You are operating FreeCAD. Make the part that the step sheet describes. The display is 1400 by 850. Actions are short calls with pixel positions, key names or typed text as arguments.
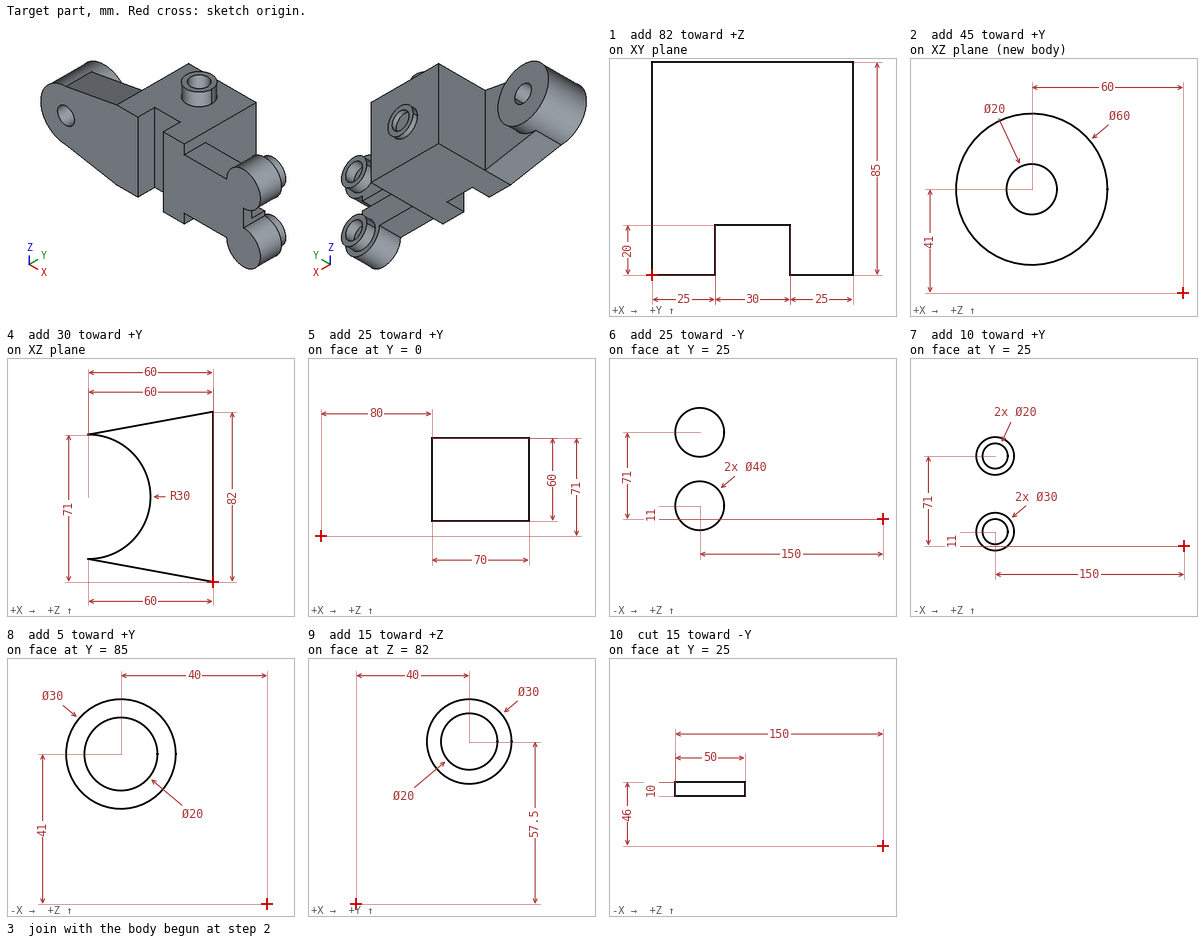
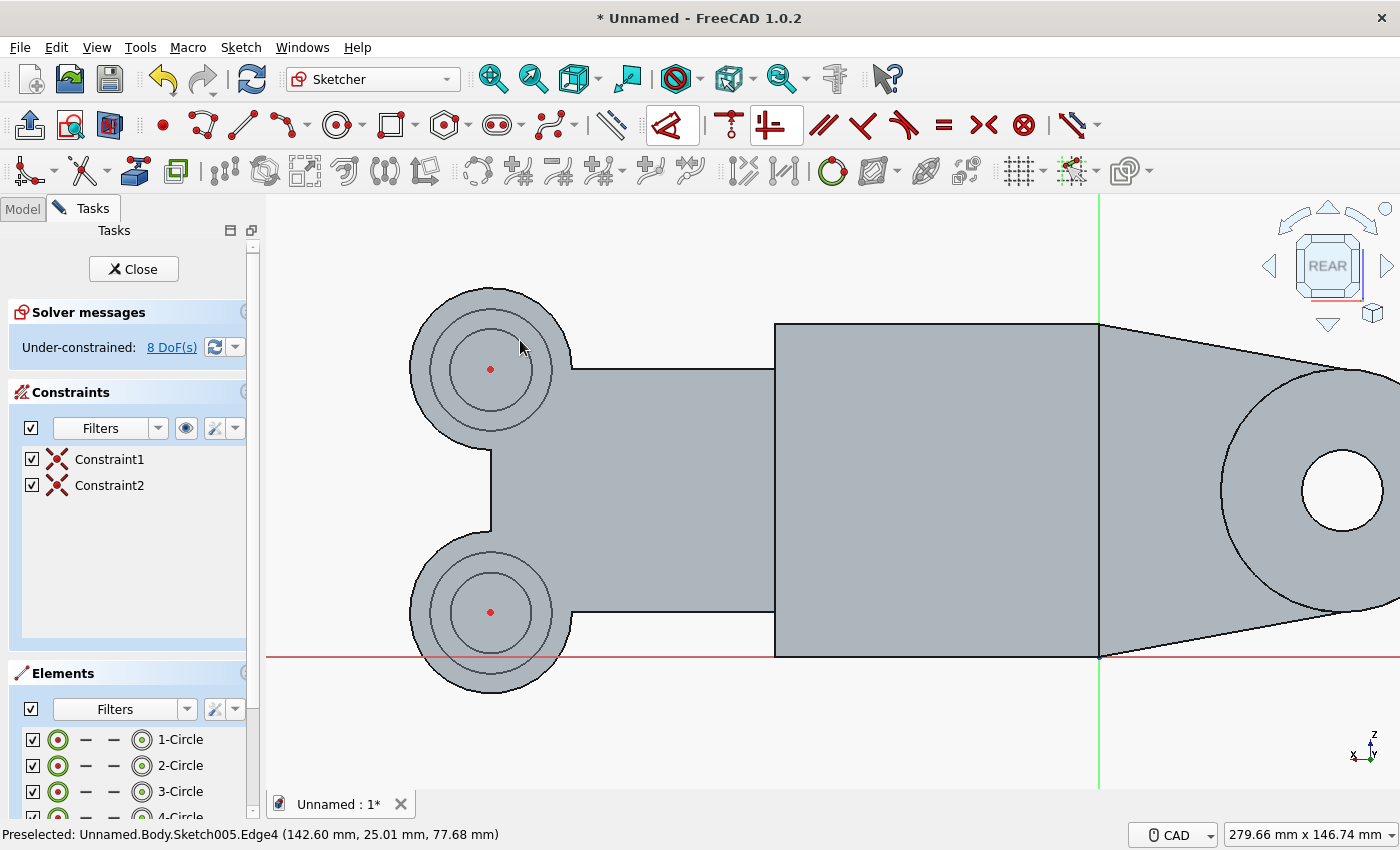
click(534, 570)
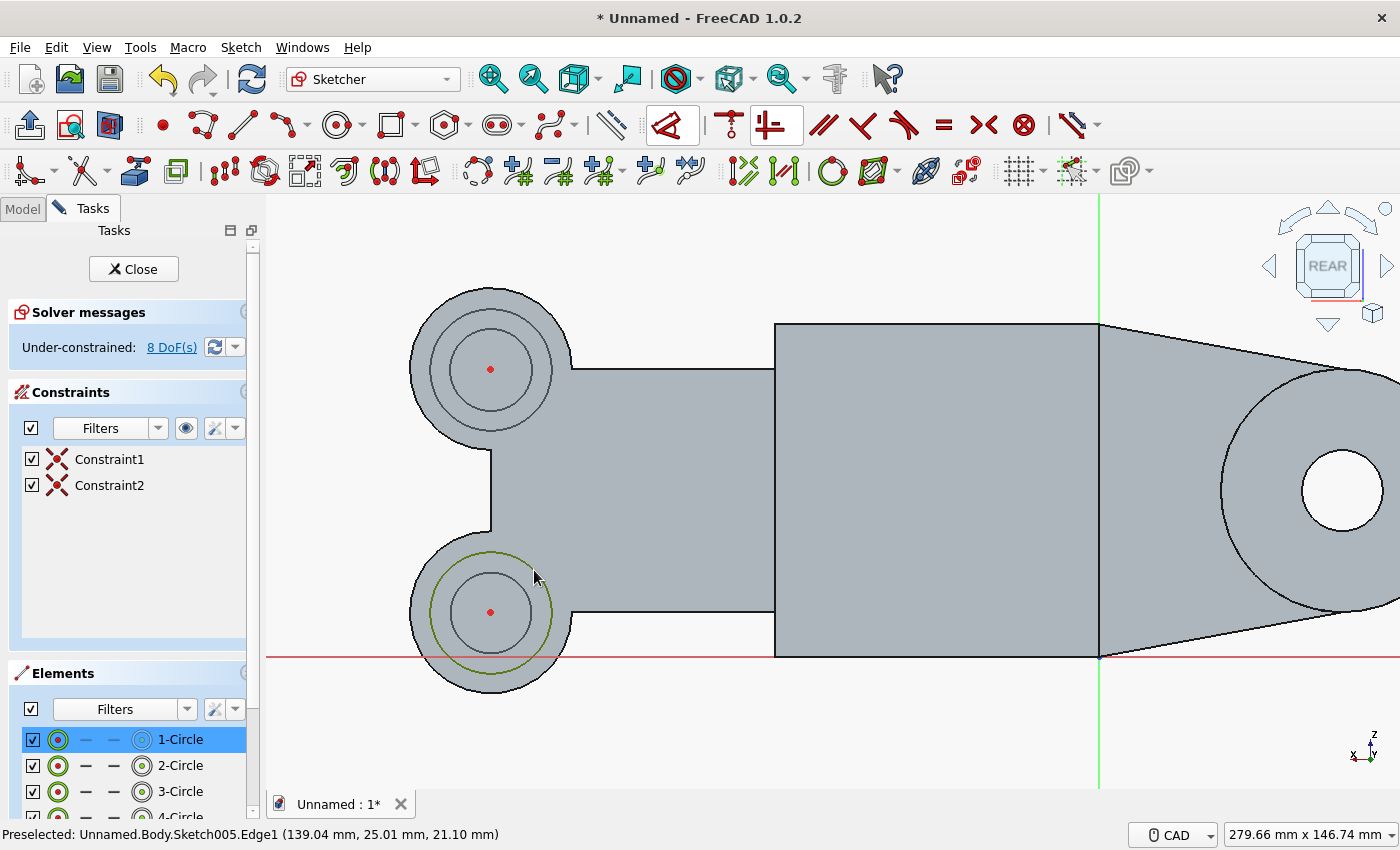
click(534, 327)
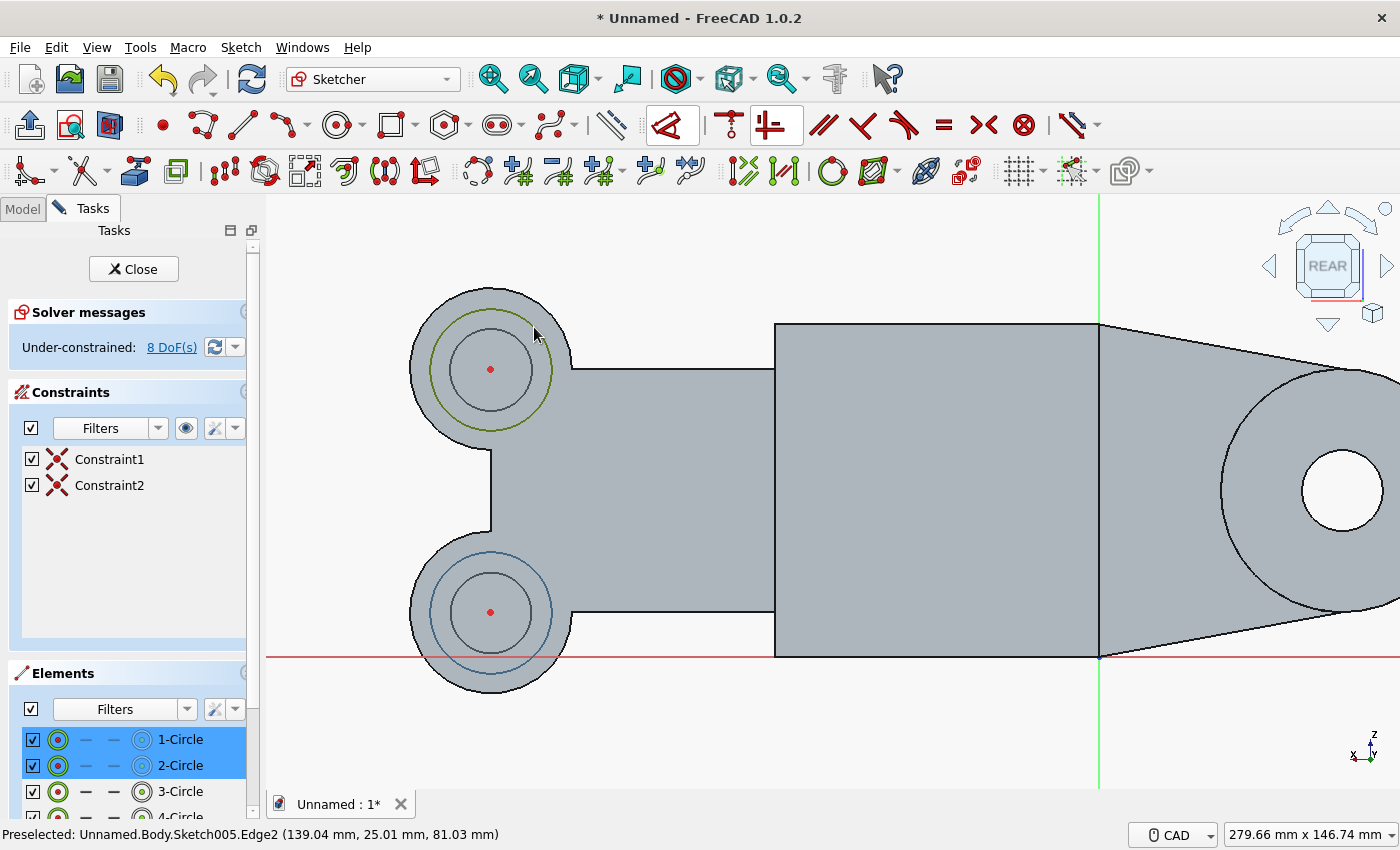
click(944, 126)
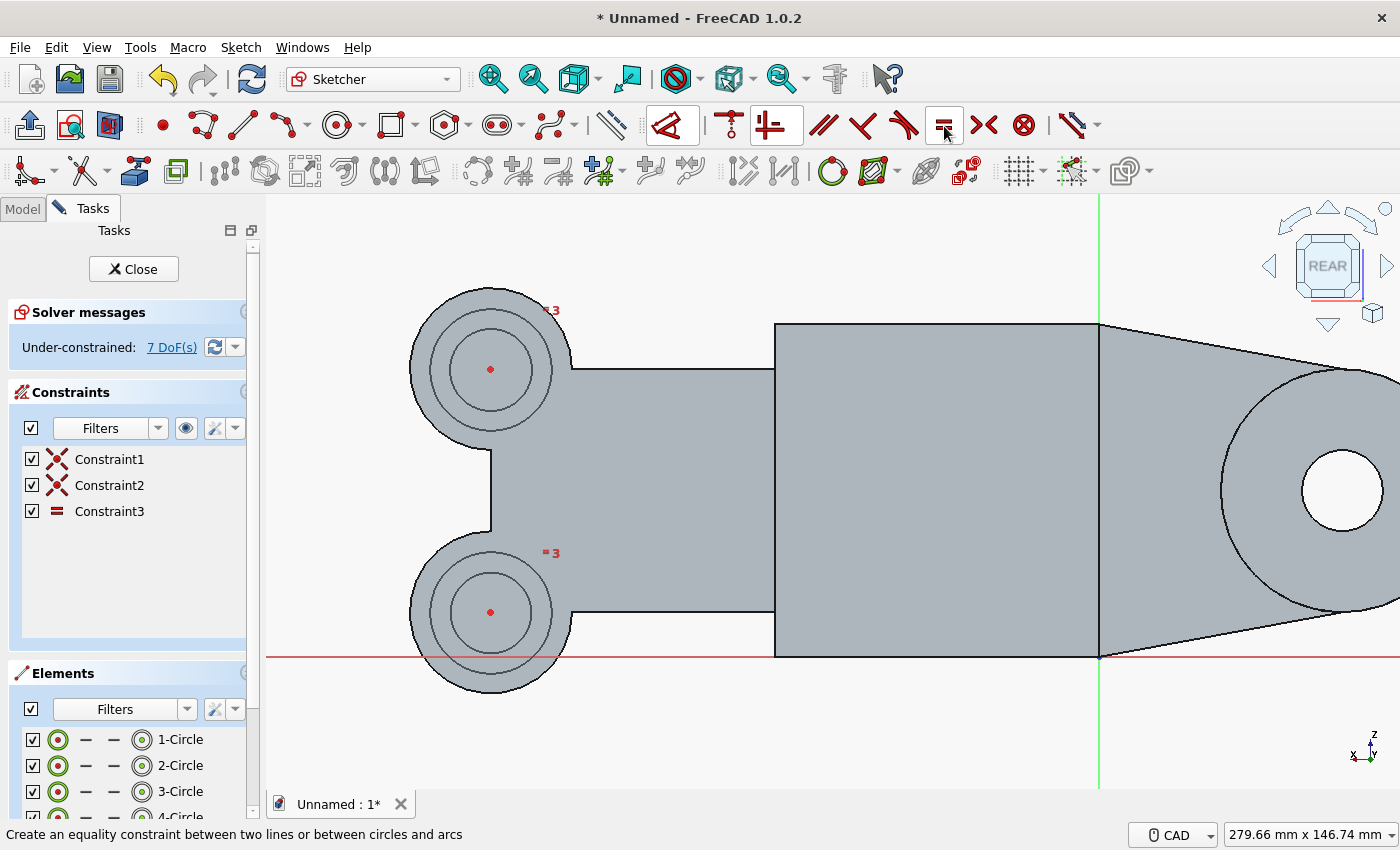
click(519, 584)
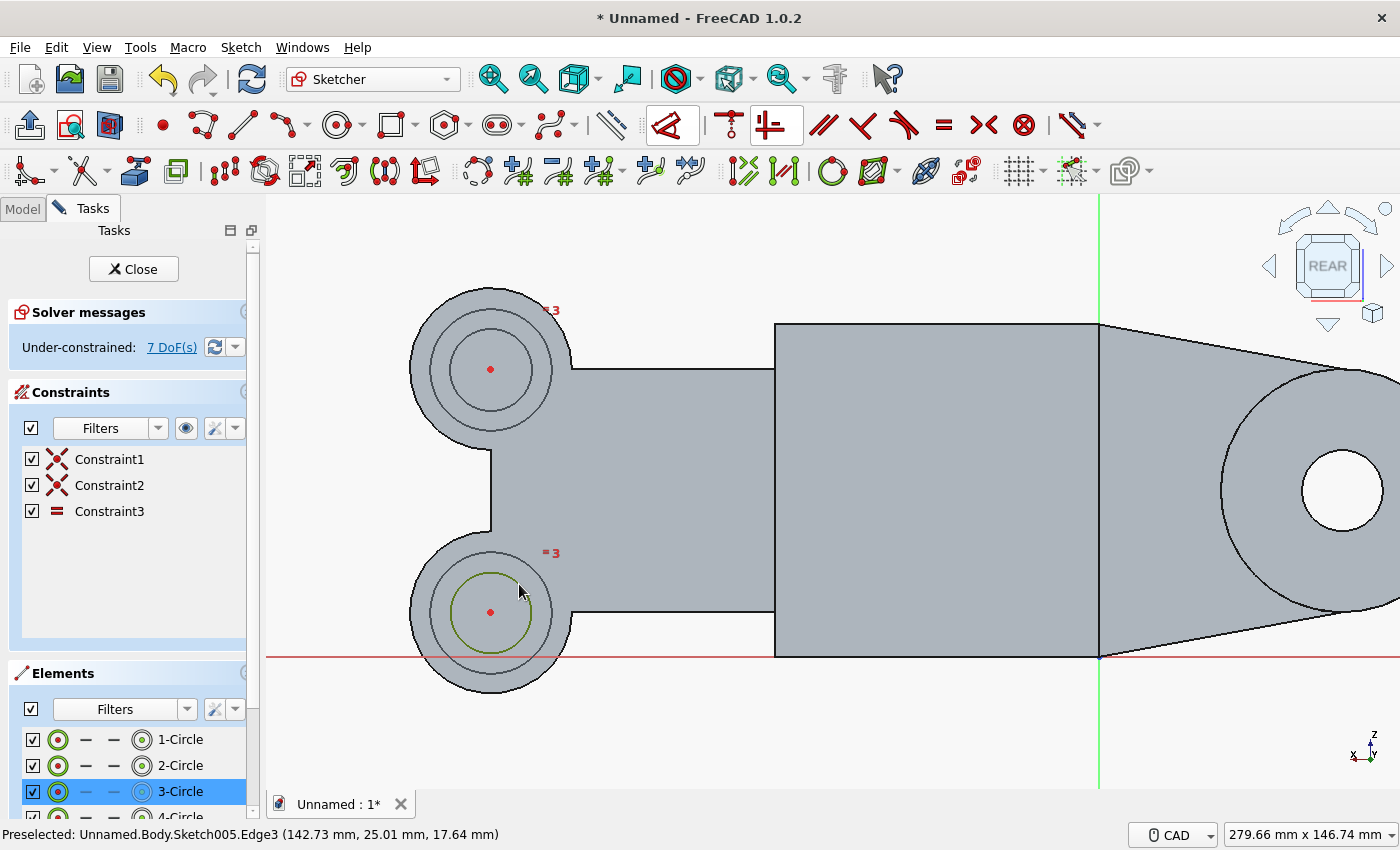
click(520, 341)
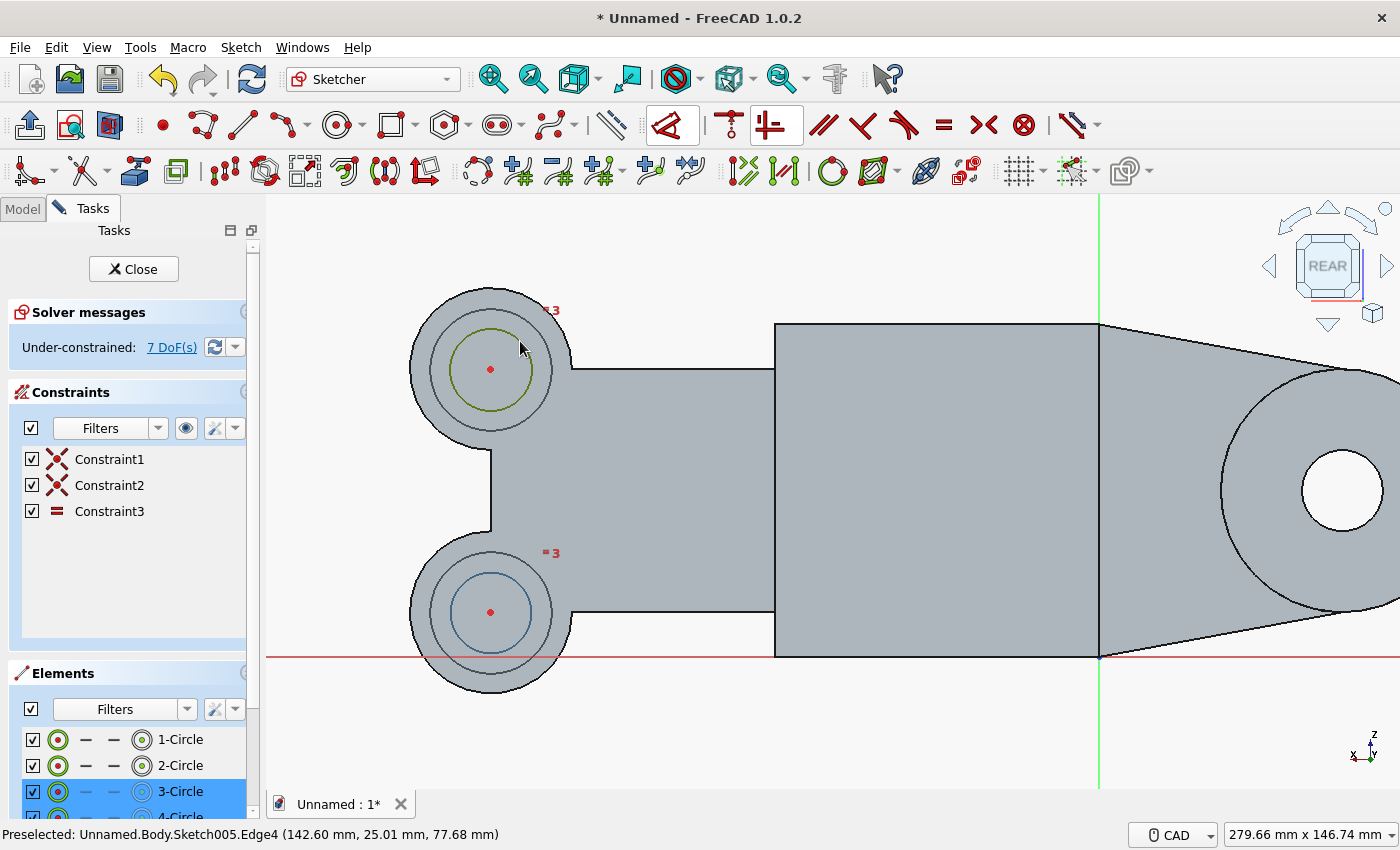
click(944, 126)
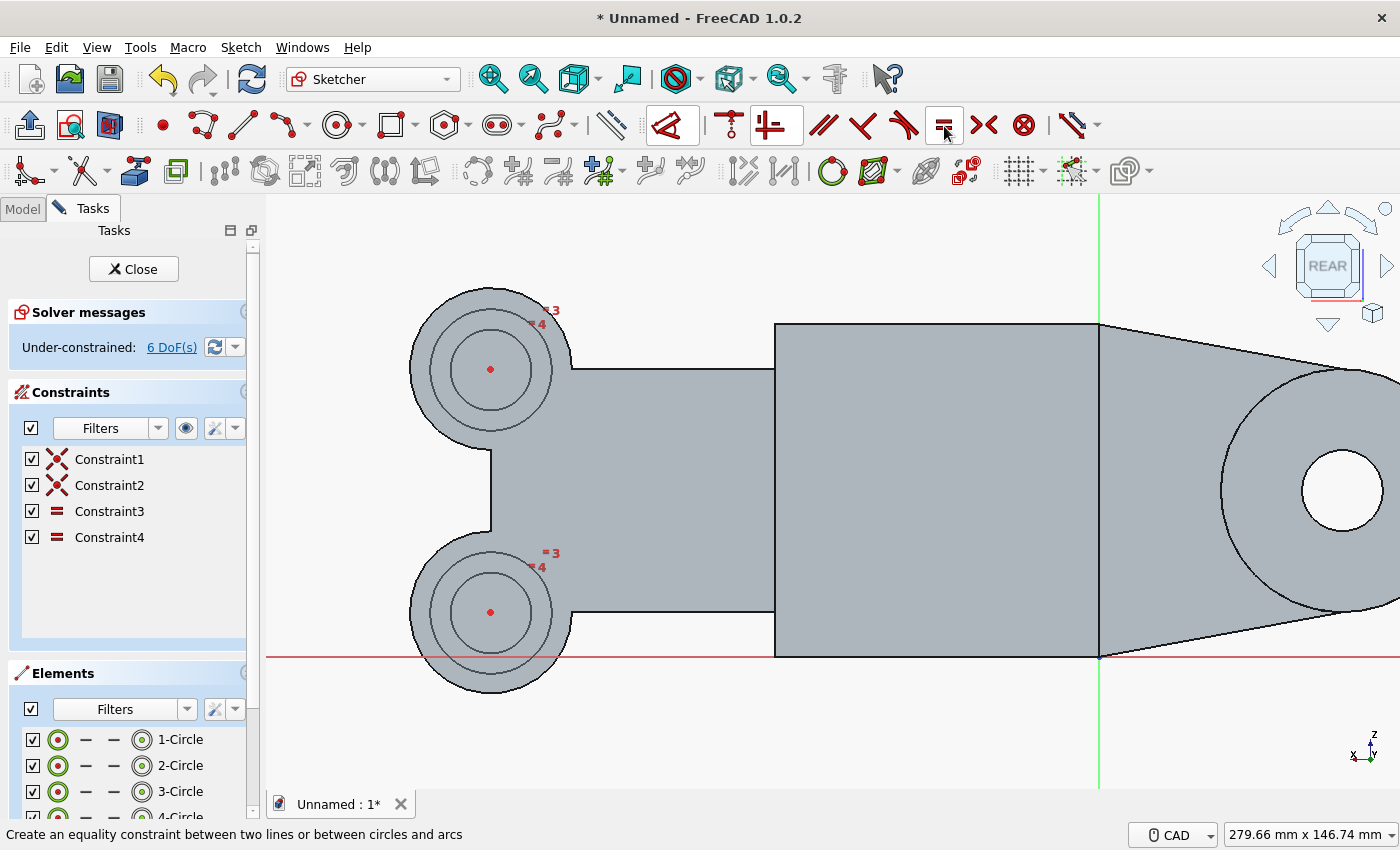
click(491, 613)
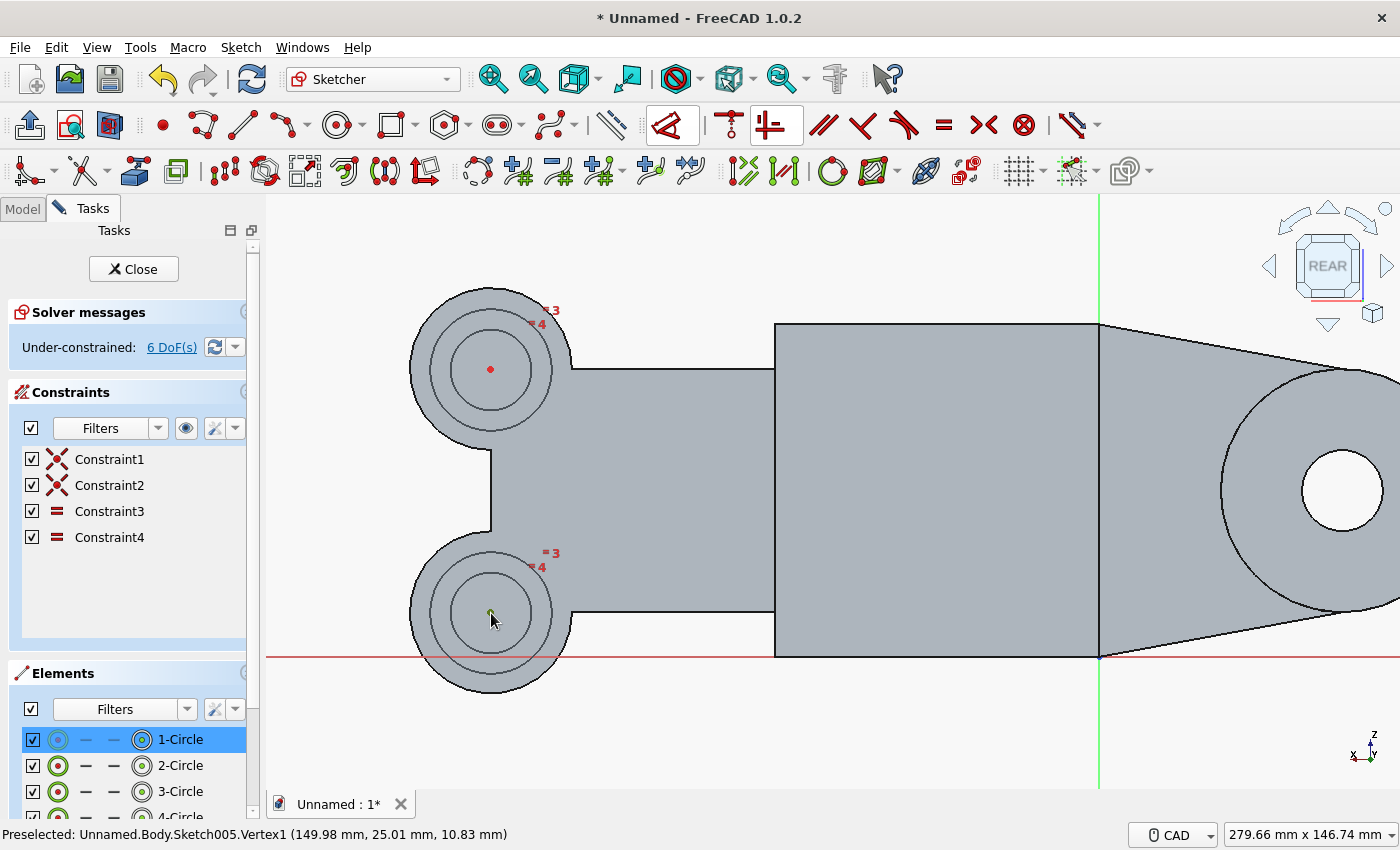
click(491, 370)